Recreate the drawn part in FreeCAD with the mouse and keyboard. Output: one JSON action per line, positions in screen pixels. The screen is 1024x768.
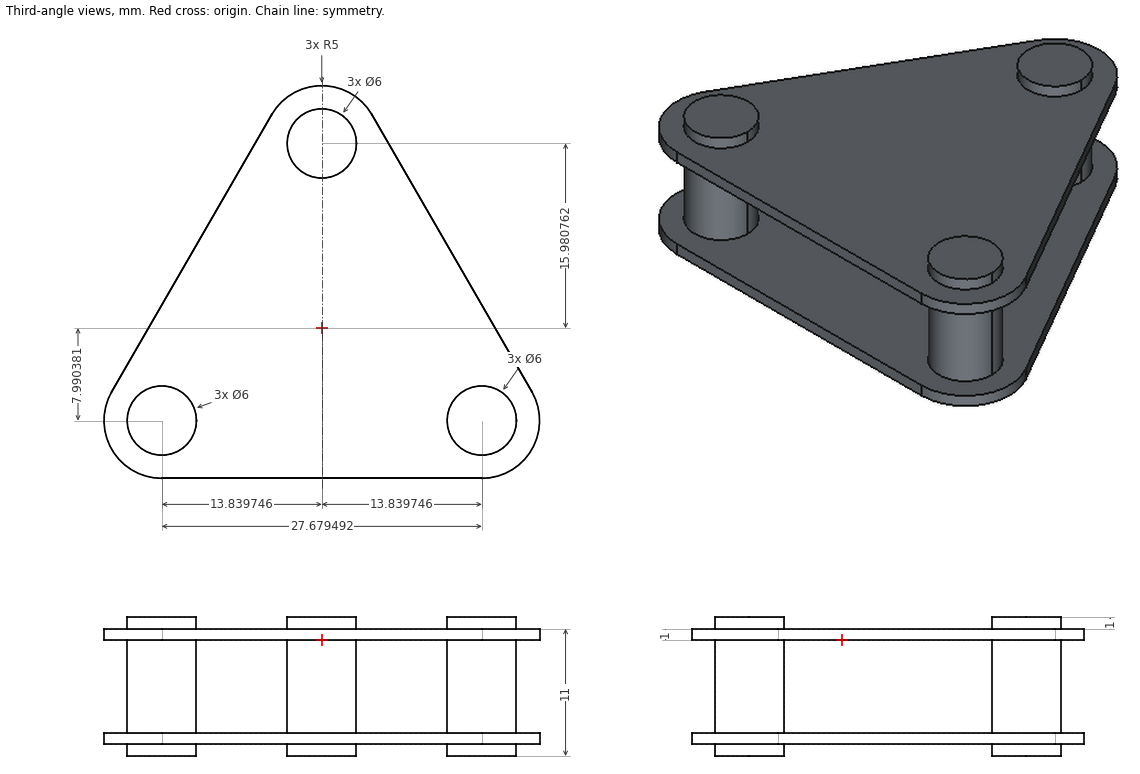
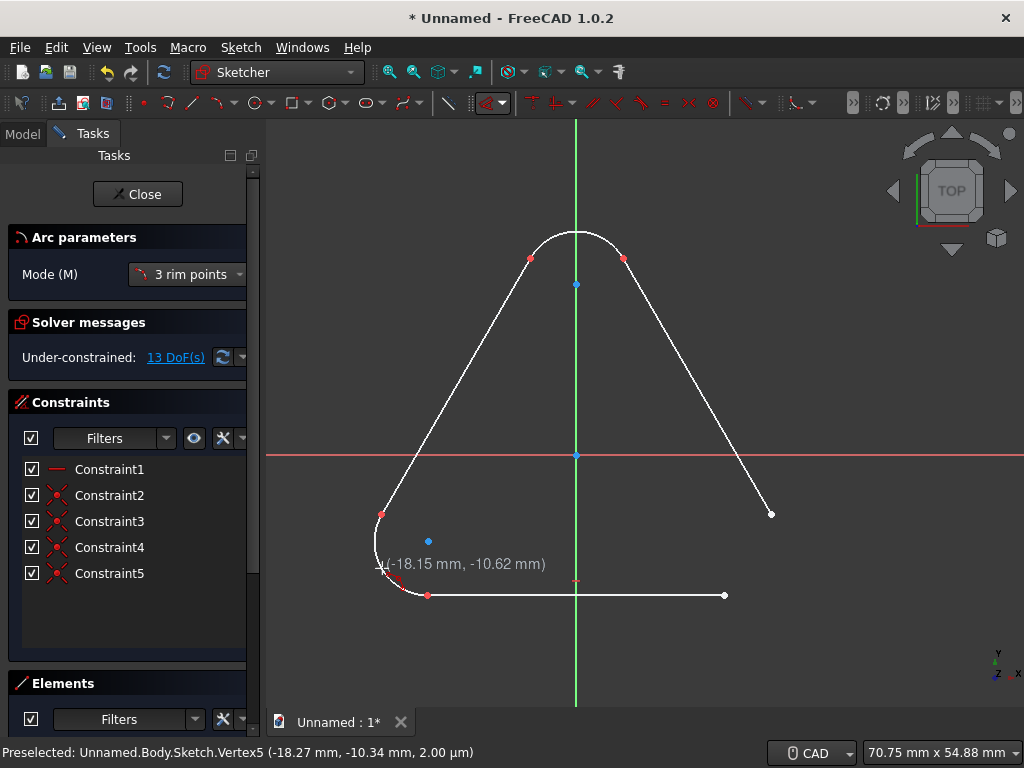
{"action": "left_click", "coordinate": [725, 595]}
{"action": "left_click", "coordinate": [772, 515]}
{"action": "left_click", "coordinate": [771, 568]}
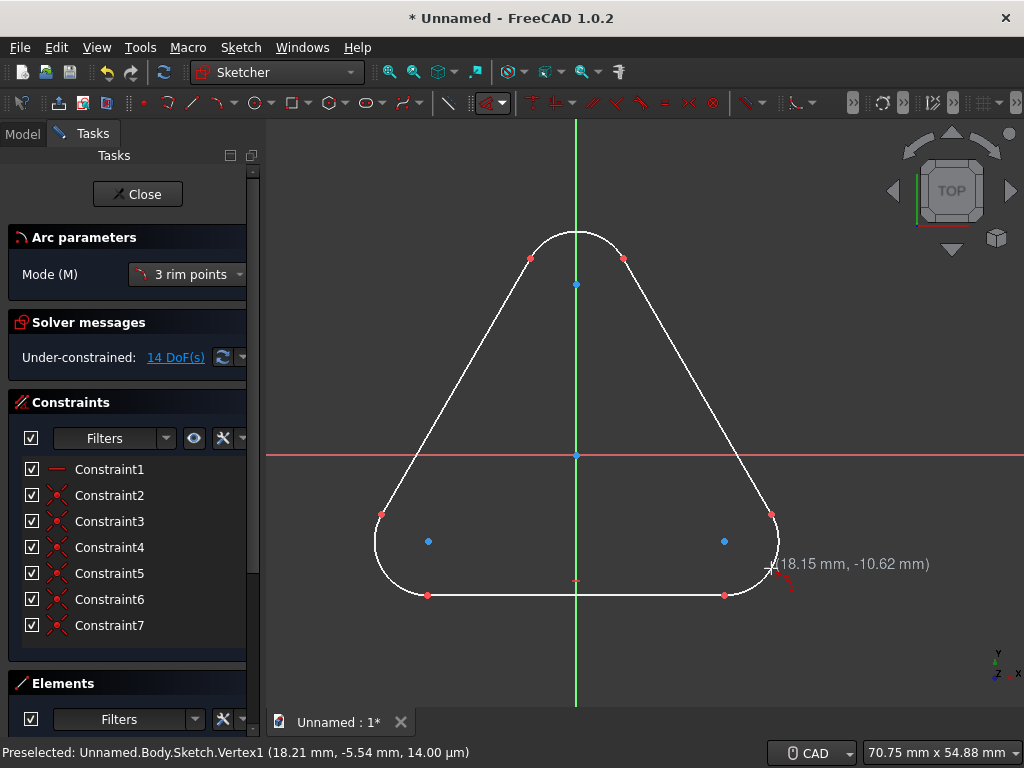
{"action": "left_click", "coordinate": [256, 104]}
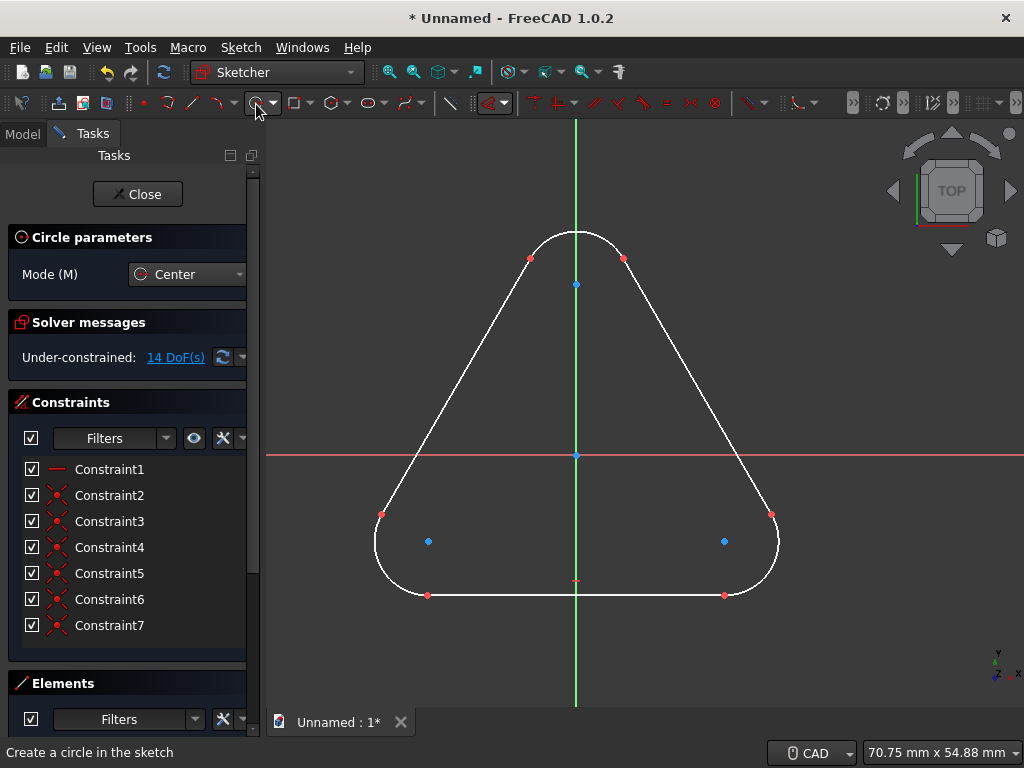
{"action": "left_click", "coordinate": [428, 541]}
{"action": "mouse_move", "coordinate": [451, 518]}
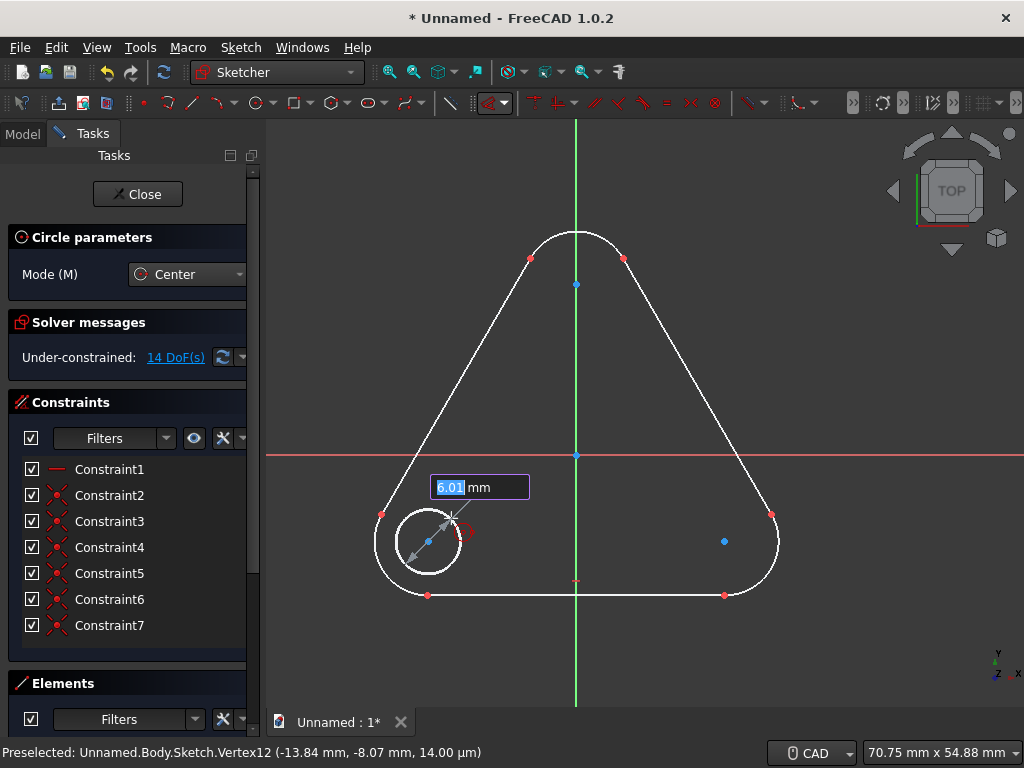
{"action": "type", "text": "6"}
{"action": "key", "text": "Return"}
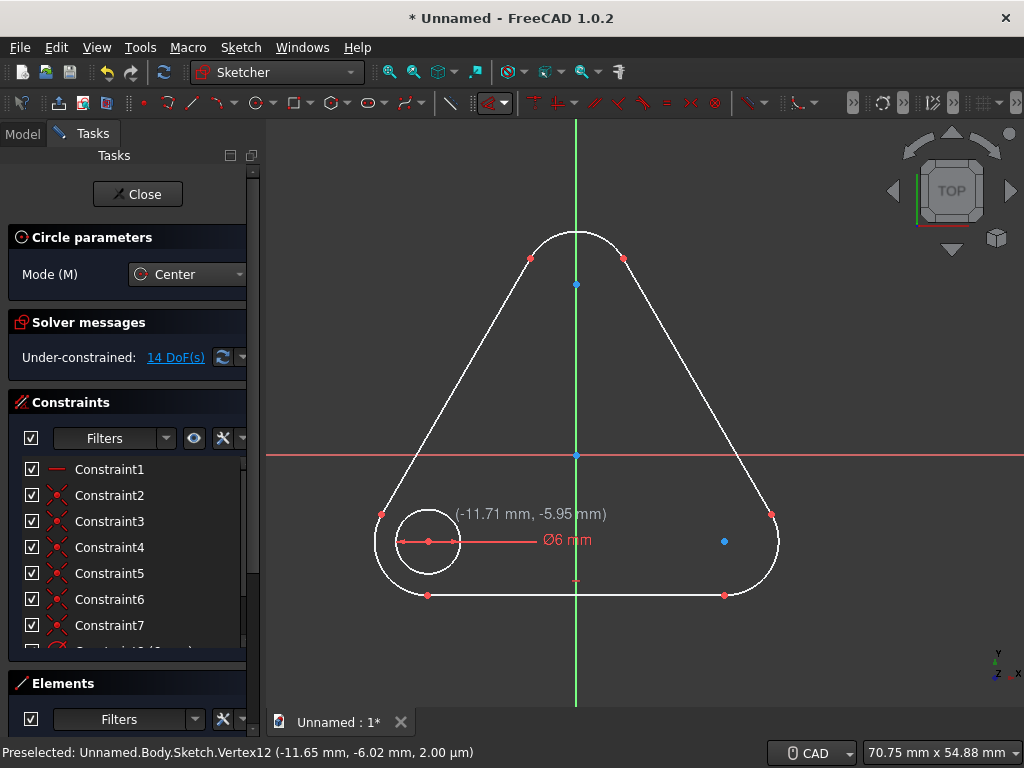
{"action": "left_click", "coordinate": [725, 541]}
{"action": "mouse_move", "coordinate": [748, 518]}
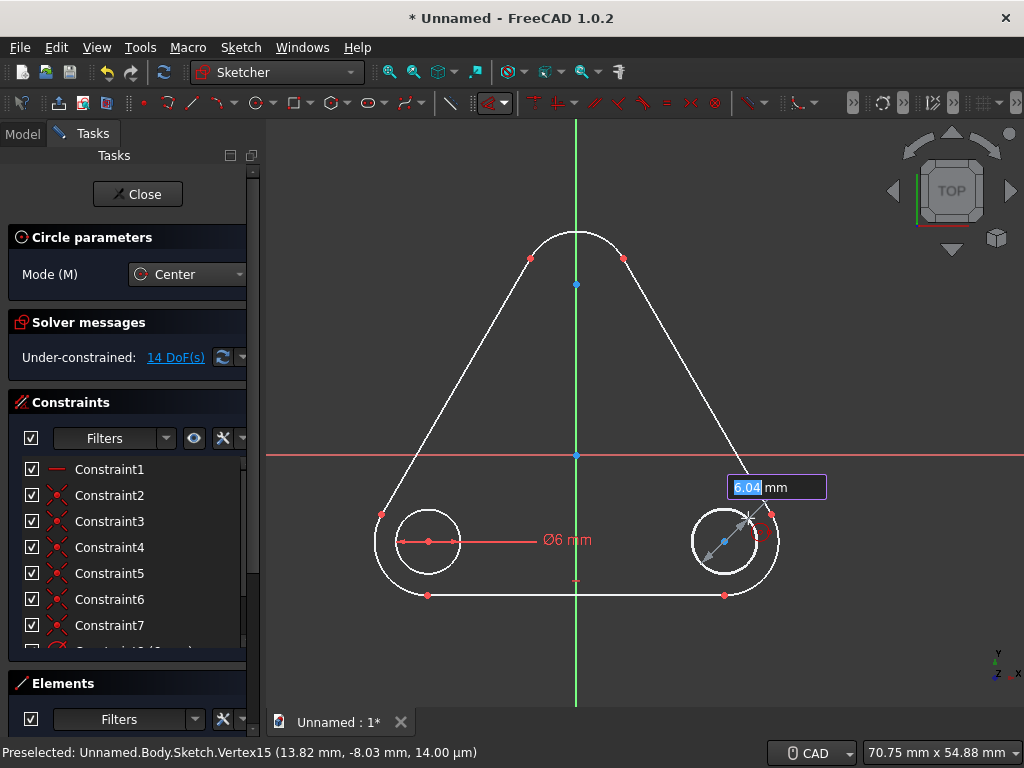
{"action": "type", "text": "6"}
{"action": "key", "text": "Return"}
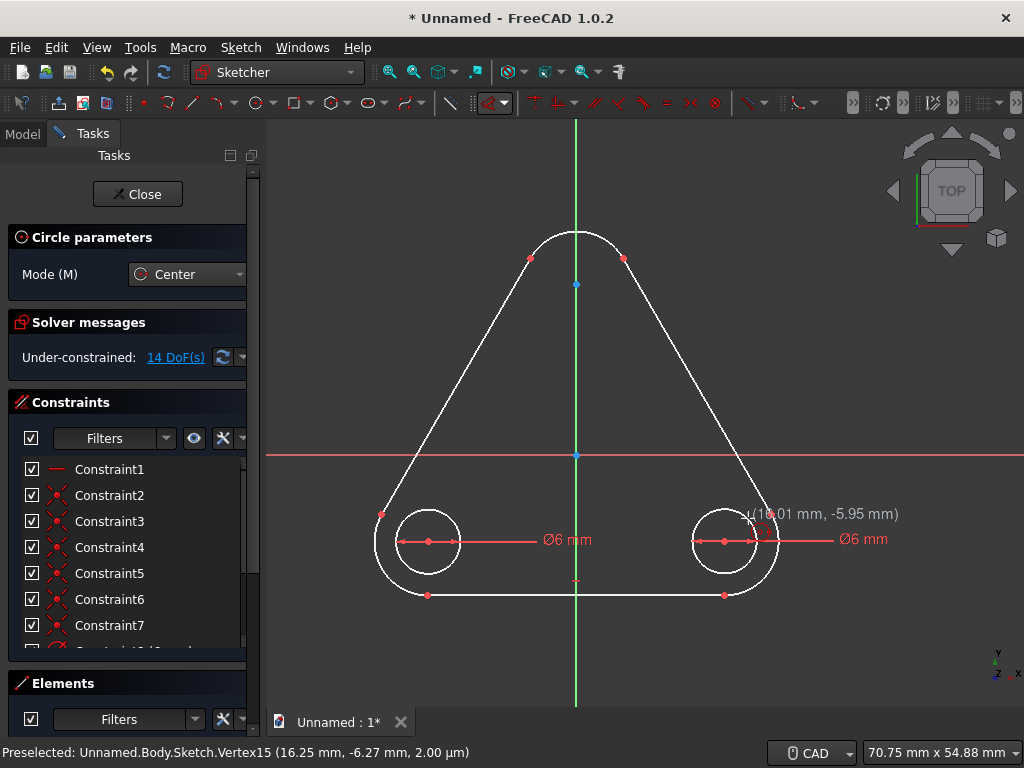
{"action": "left_click", "coordinate": [576, 284]}
{"action": "mouse_move", "coordinate": [599, 261]}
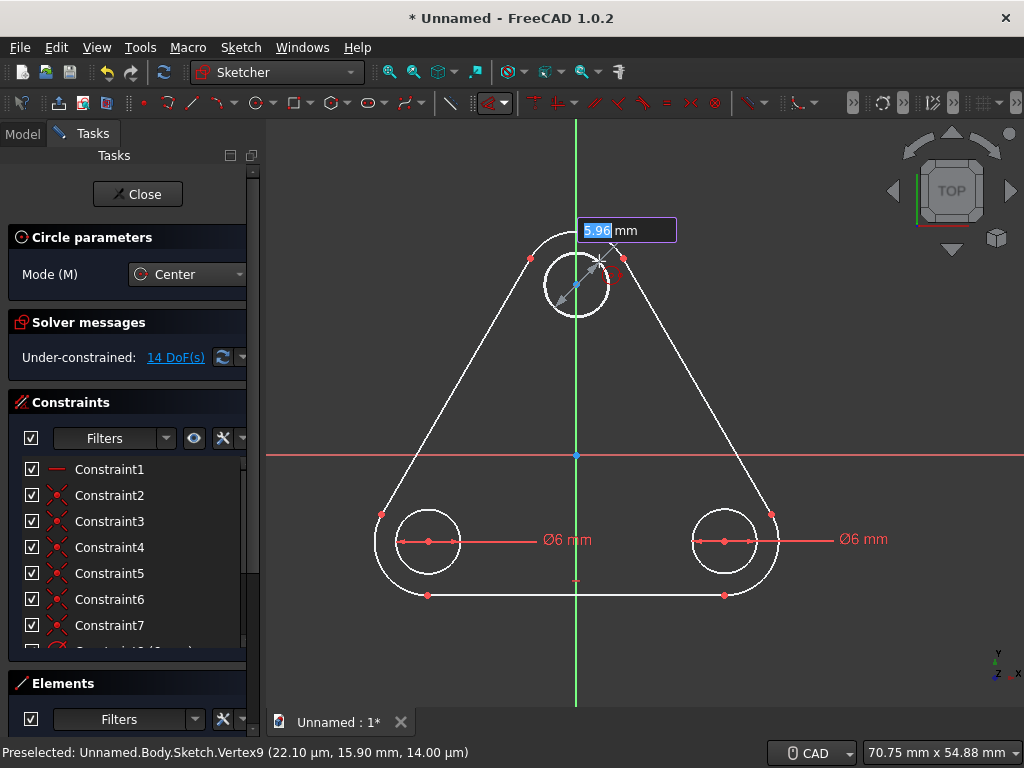
{"action": "type", "text": "6"}
{"action": "key", "text": "Return"}
{"action": "key", "text": "Escape"}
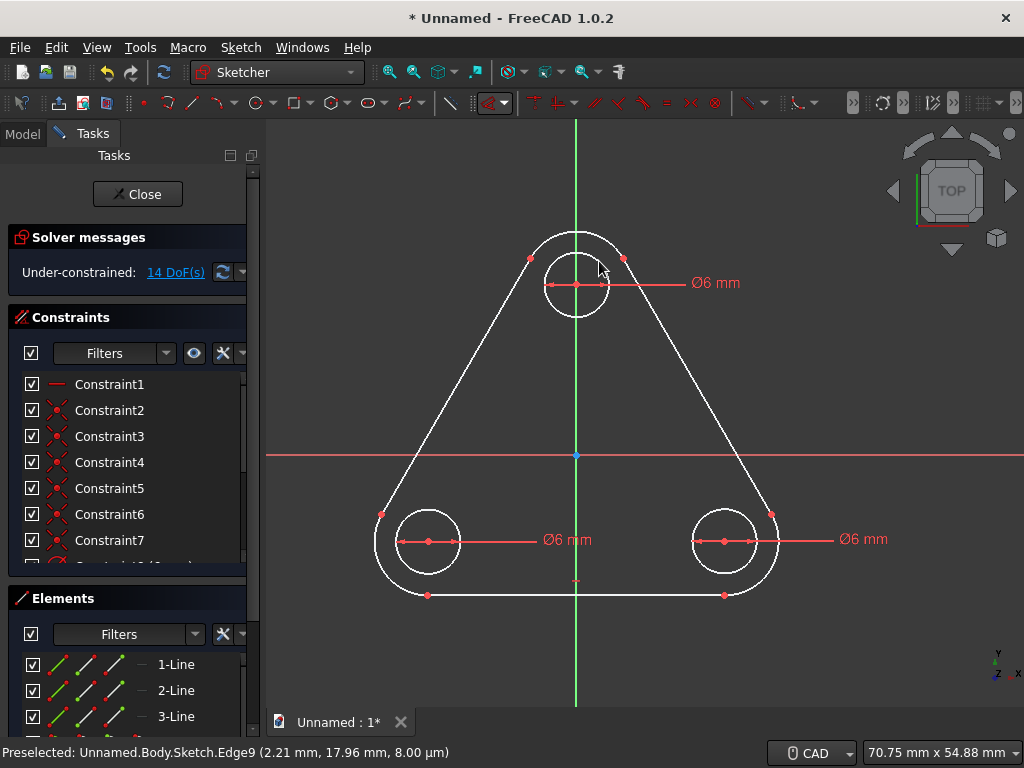
{"action": "left_click", "coordinate": [727, 438]}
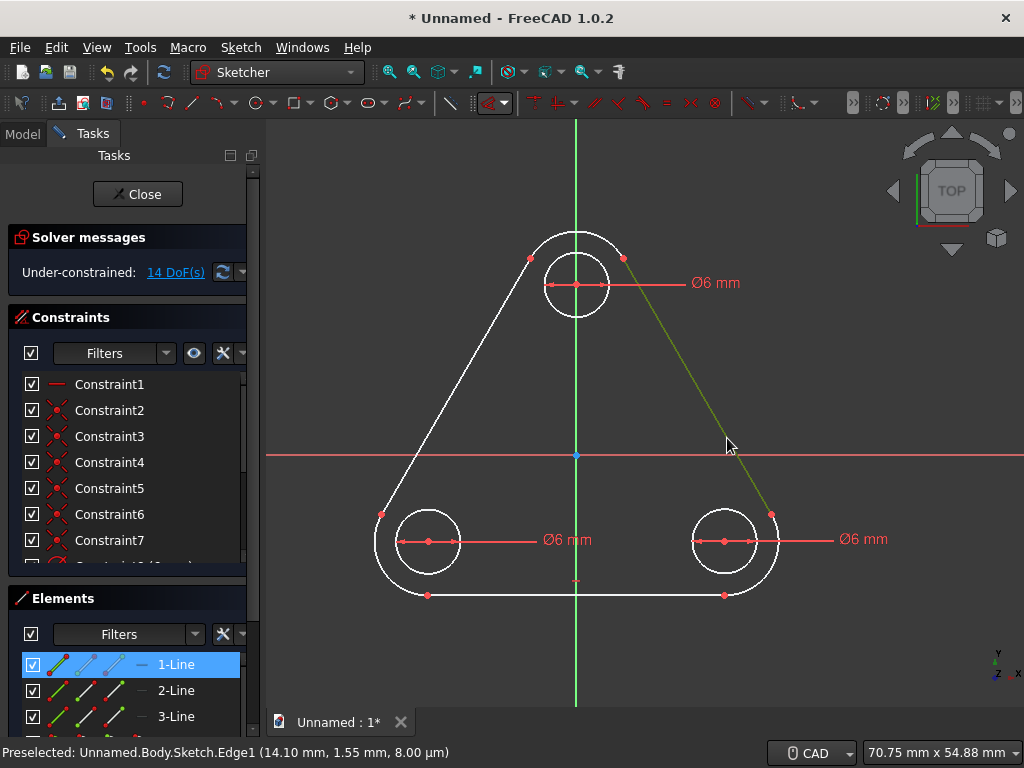
{"action": "left_click", "coordinate": [599, 236]}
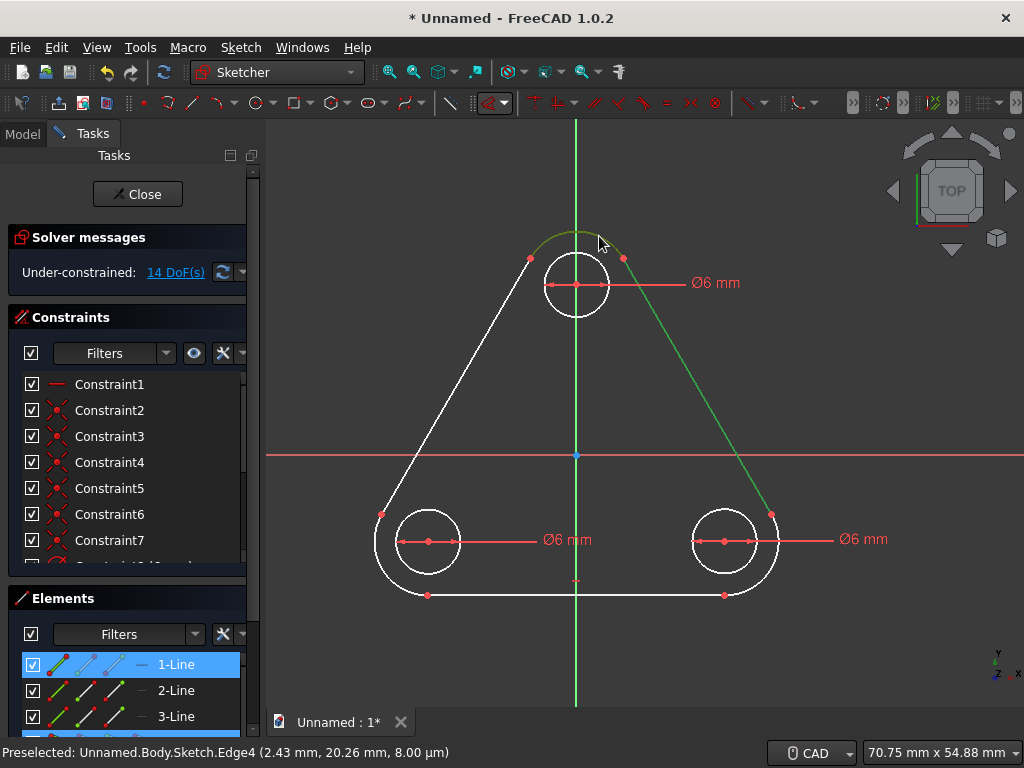
{"action": "left_click", "coordinate": [644, 104]}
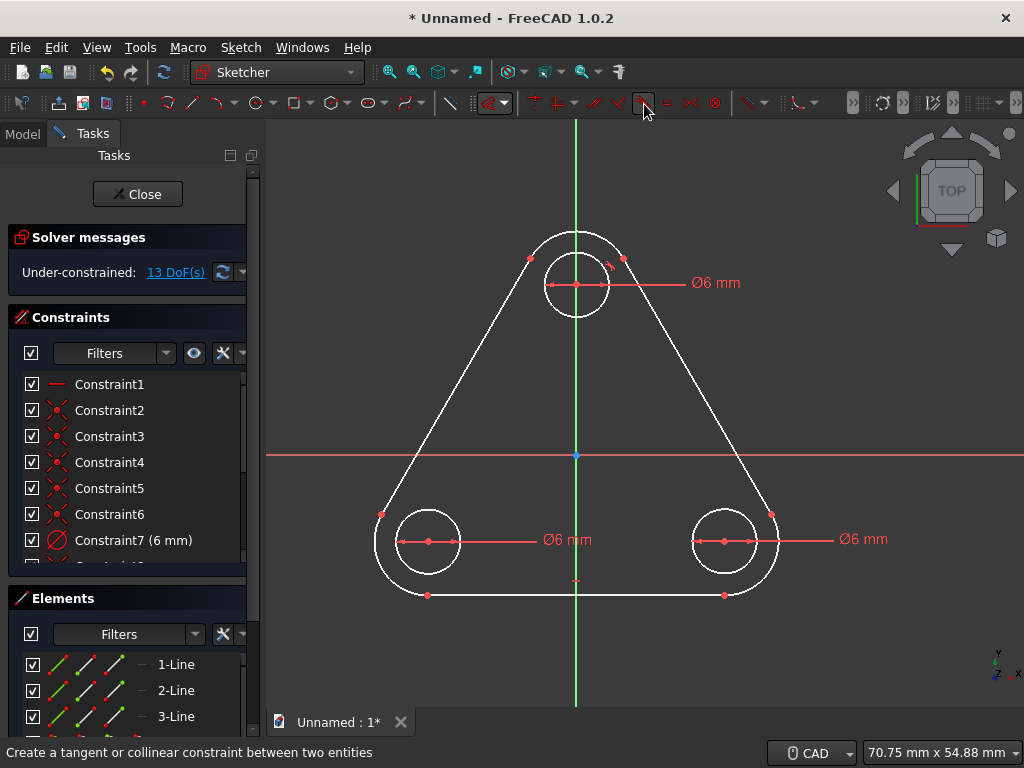
{"action": "left_click", "coordinate": [727, 438]}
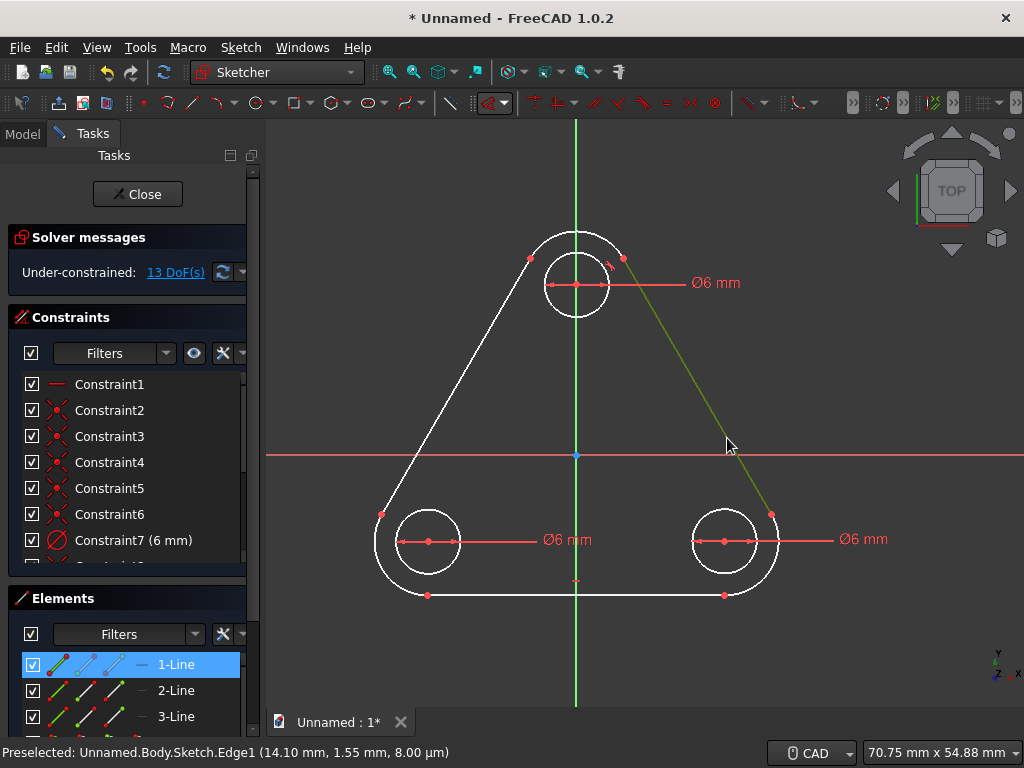
{"action": "left_click", "coordinate": [756, 585]}